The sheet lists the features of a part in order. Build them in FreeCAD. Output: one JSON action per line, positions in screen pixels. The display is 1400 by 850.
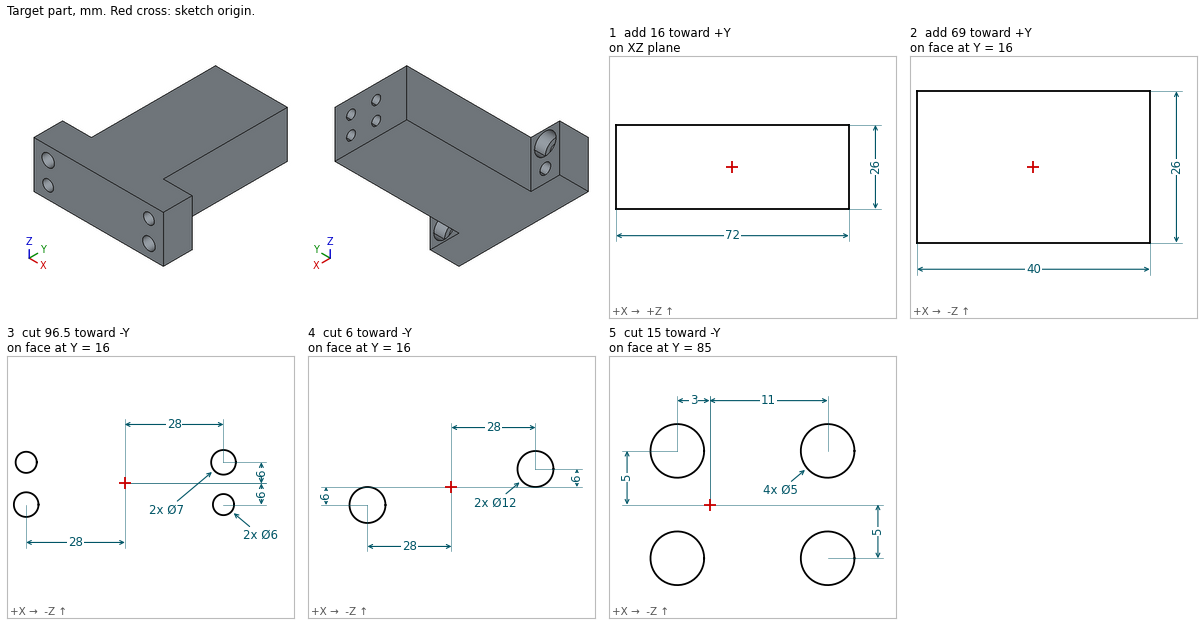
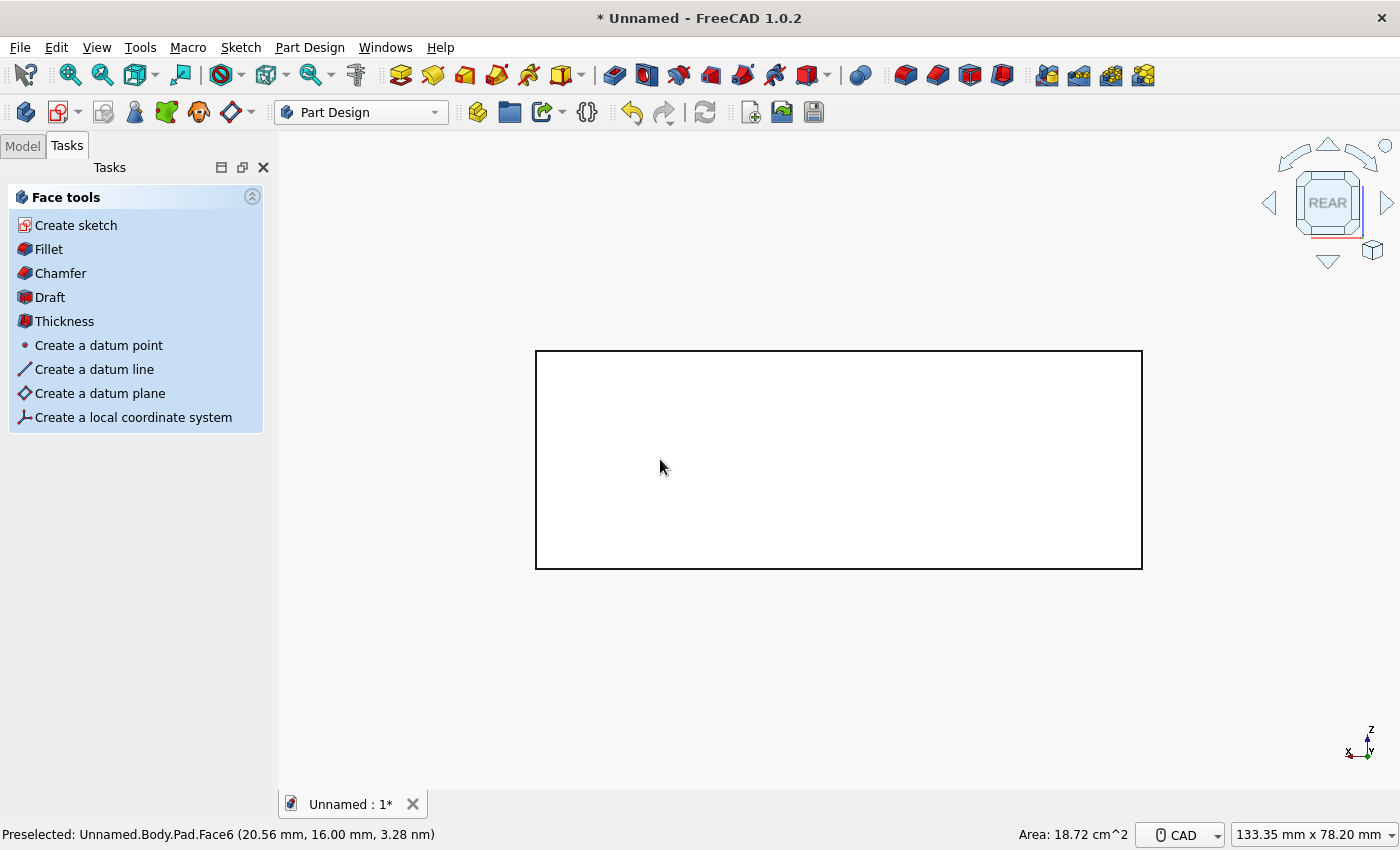
{"action": "left_click", "coordinate": [58, 112]}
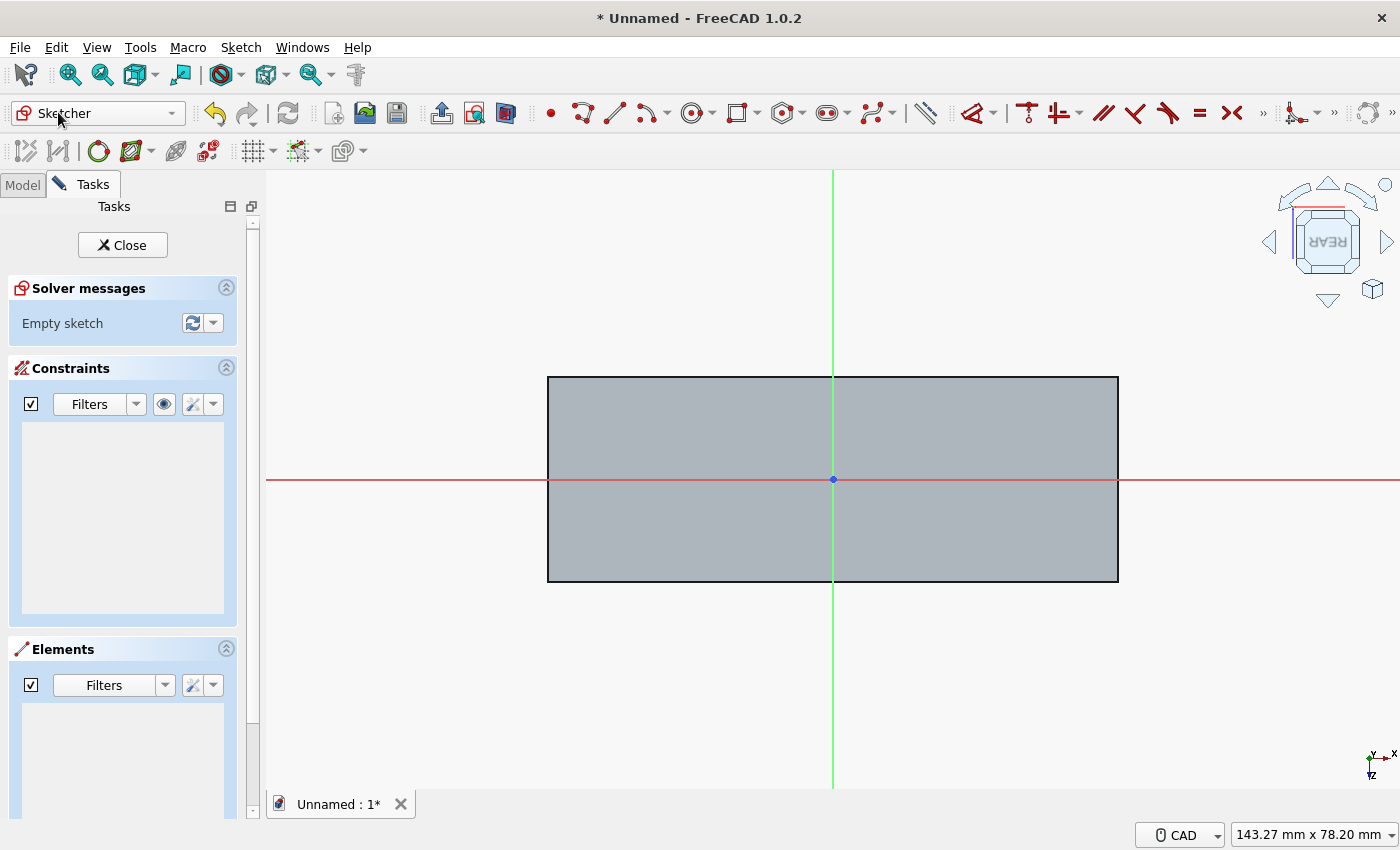
{"action": "scroll", "coordinate": [916, 479], "scroll_direction": "up", "scroll_amount": 3}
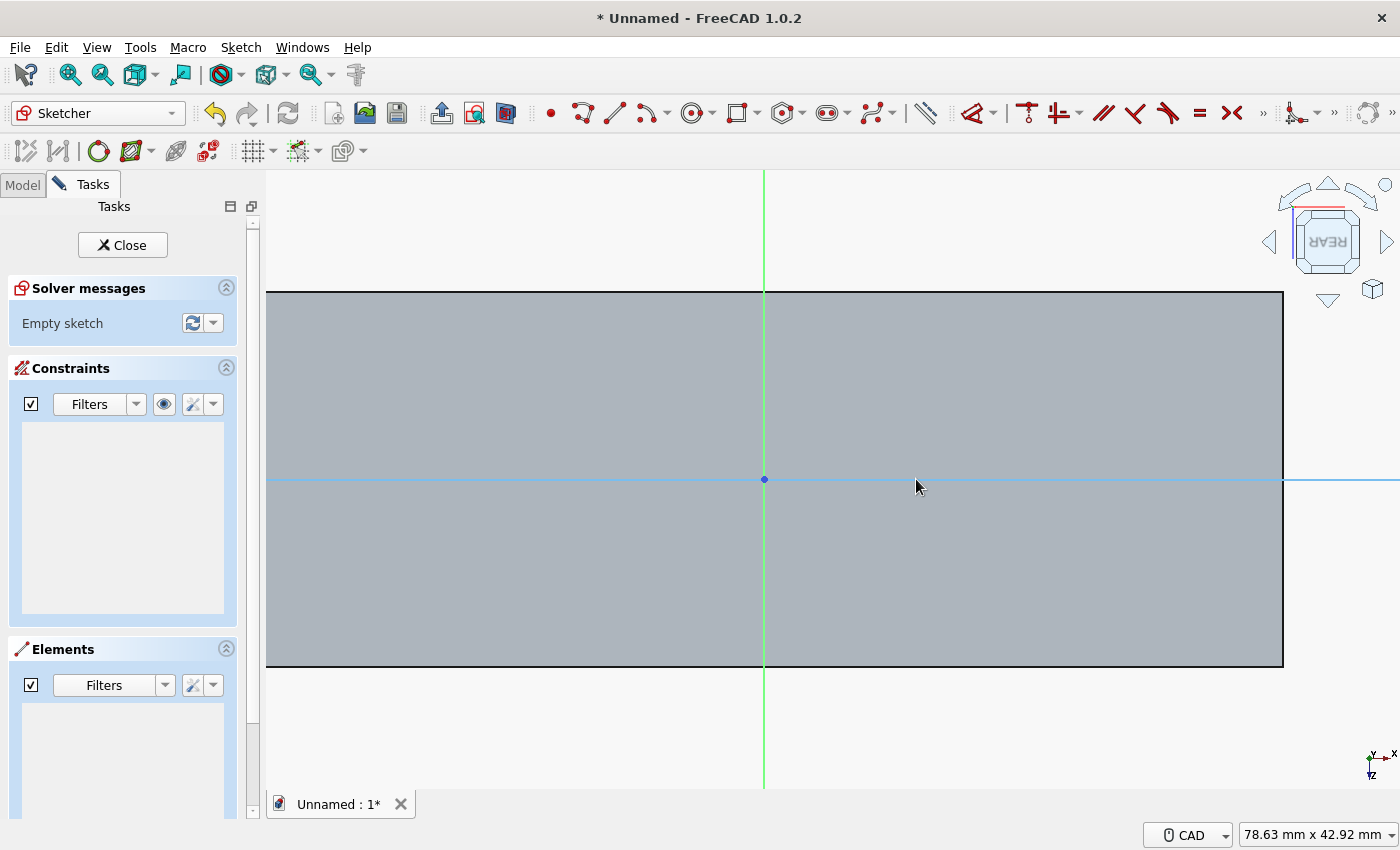
{"action": "key", "text": "g v"}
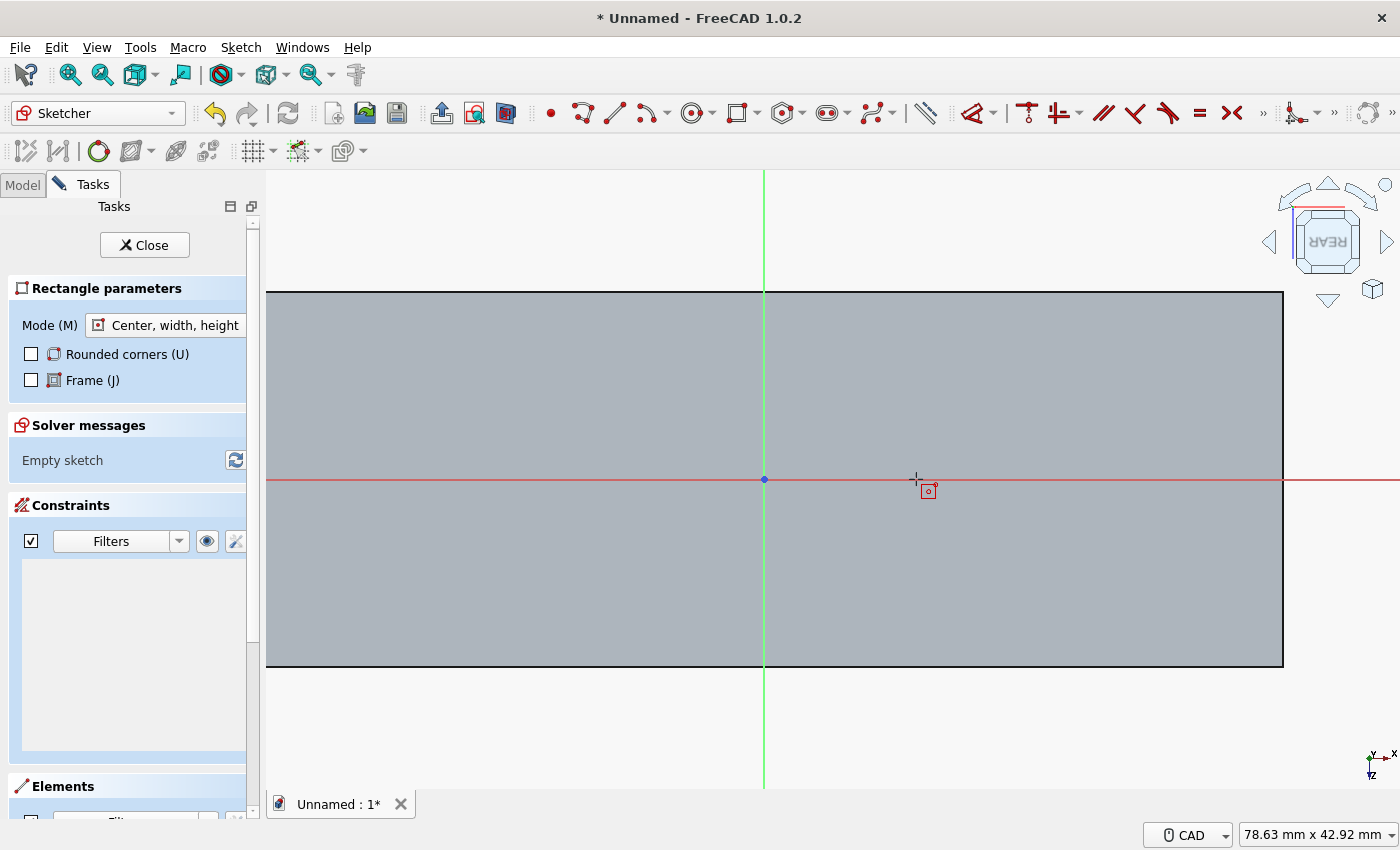
{"action": "left_click", "coordinate": [764, 479]}
{"action": "mouse_move", "coordinate": [1053, 292]}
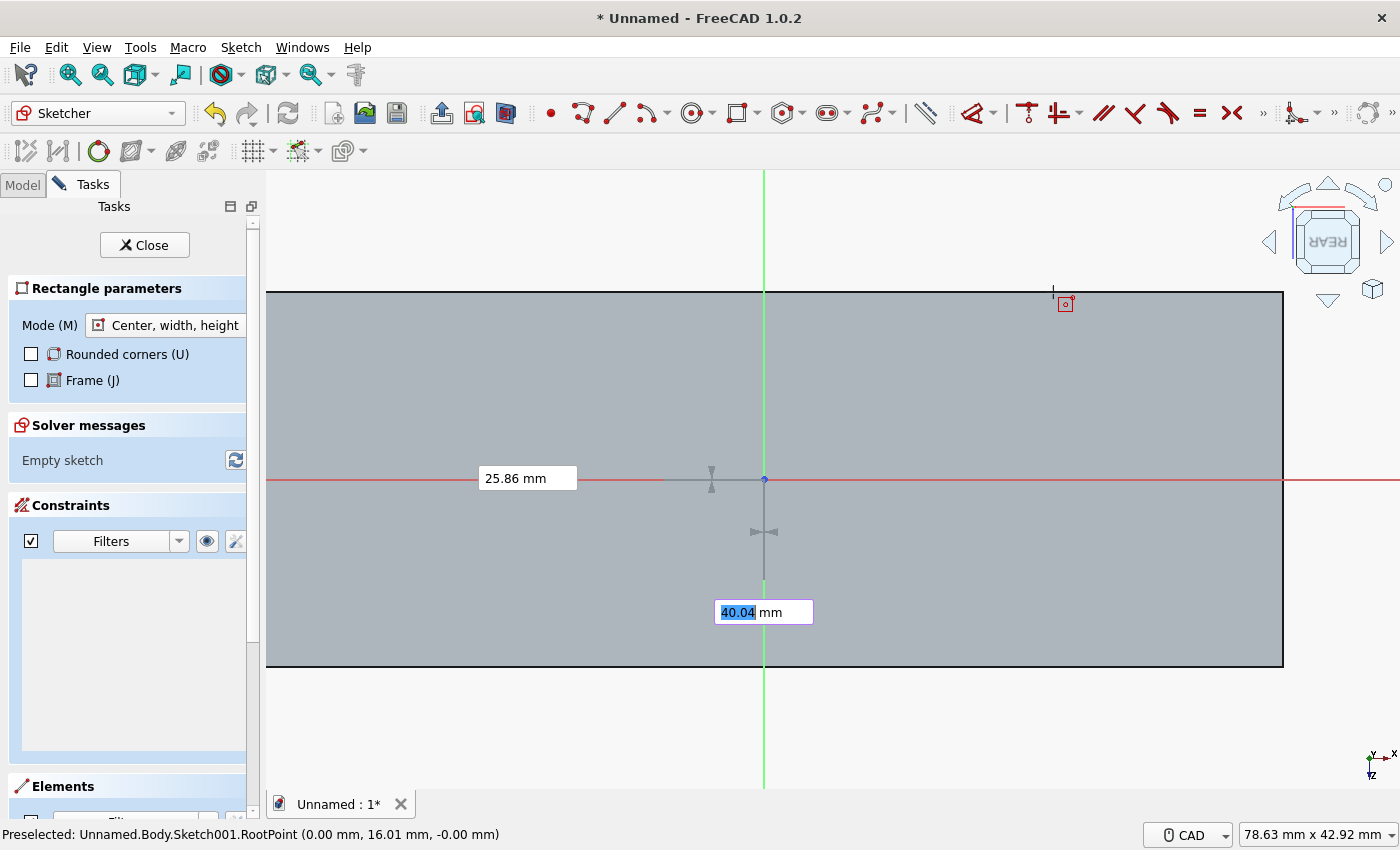
{"action": "type", "text": "40"}
{"action": "key", "text": "Tab"}
{"action": "type", "text": "26"}
{"action": "key", "text": "Return"}
{"action": "key", "text": "Escape"}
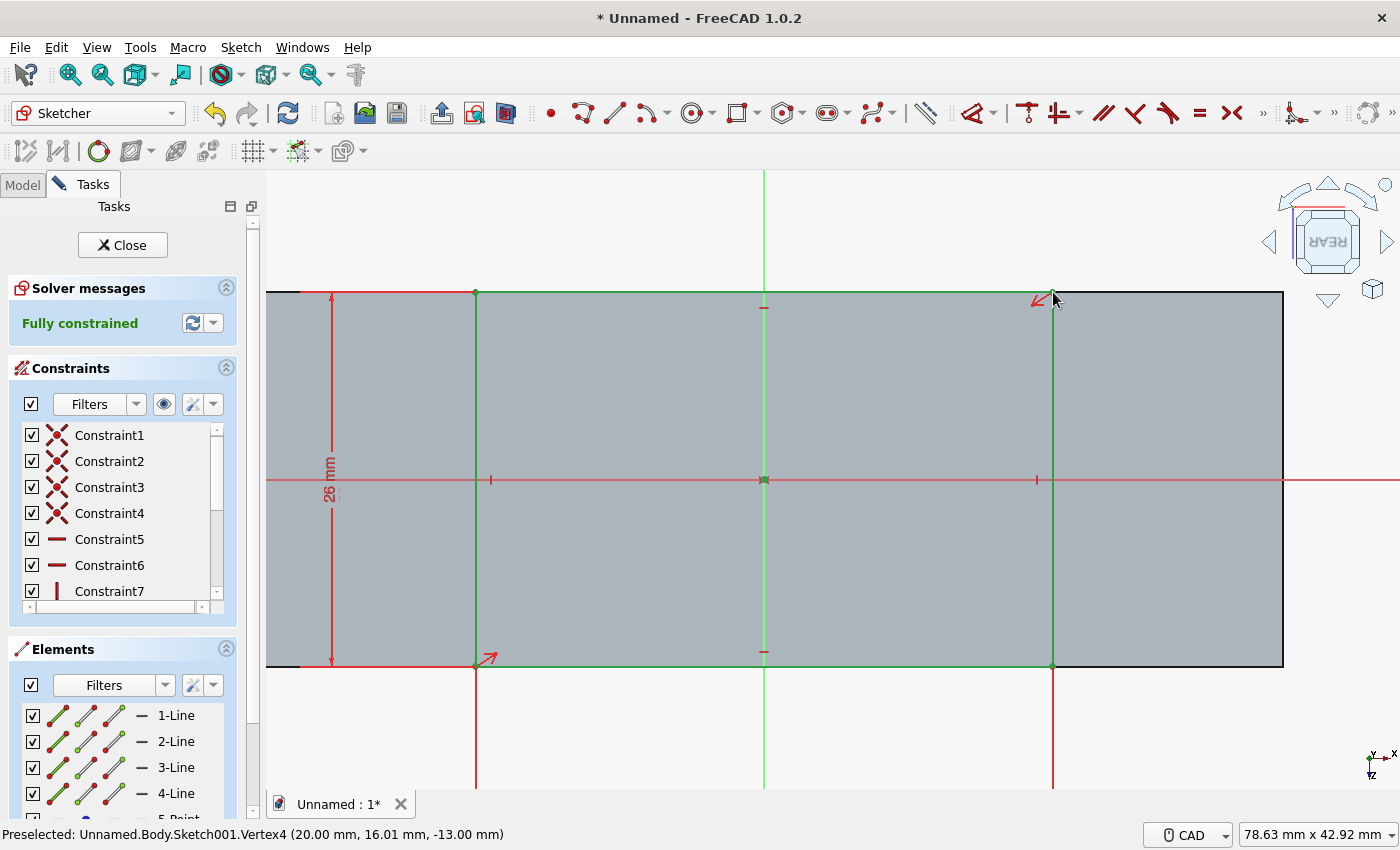
{"action": "left_click", "coordinate": [123, 245]}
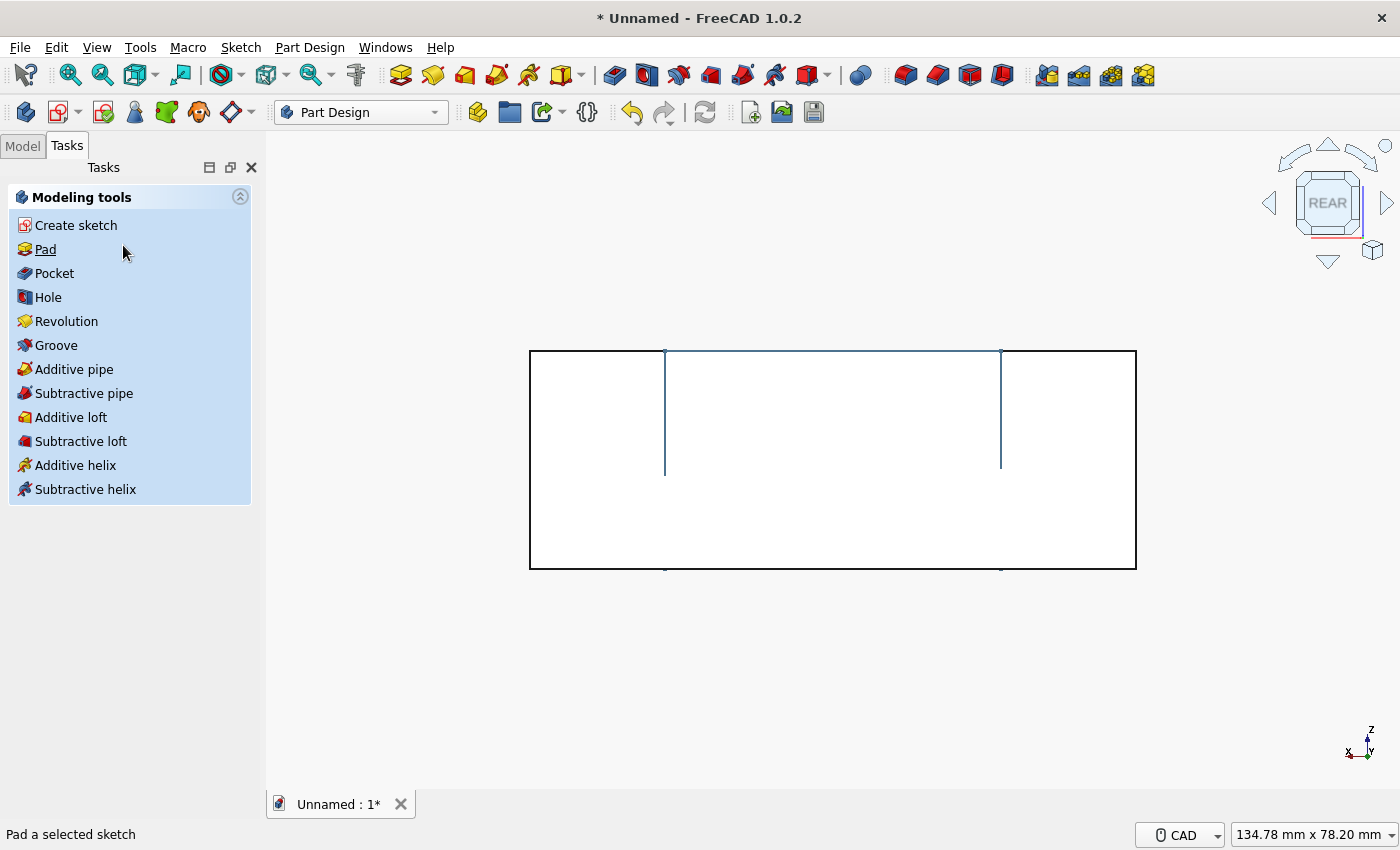
{"action": "left_click", "coordinate": [402, 76]}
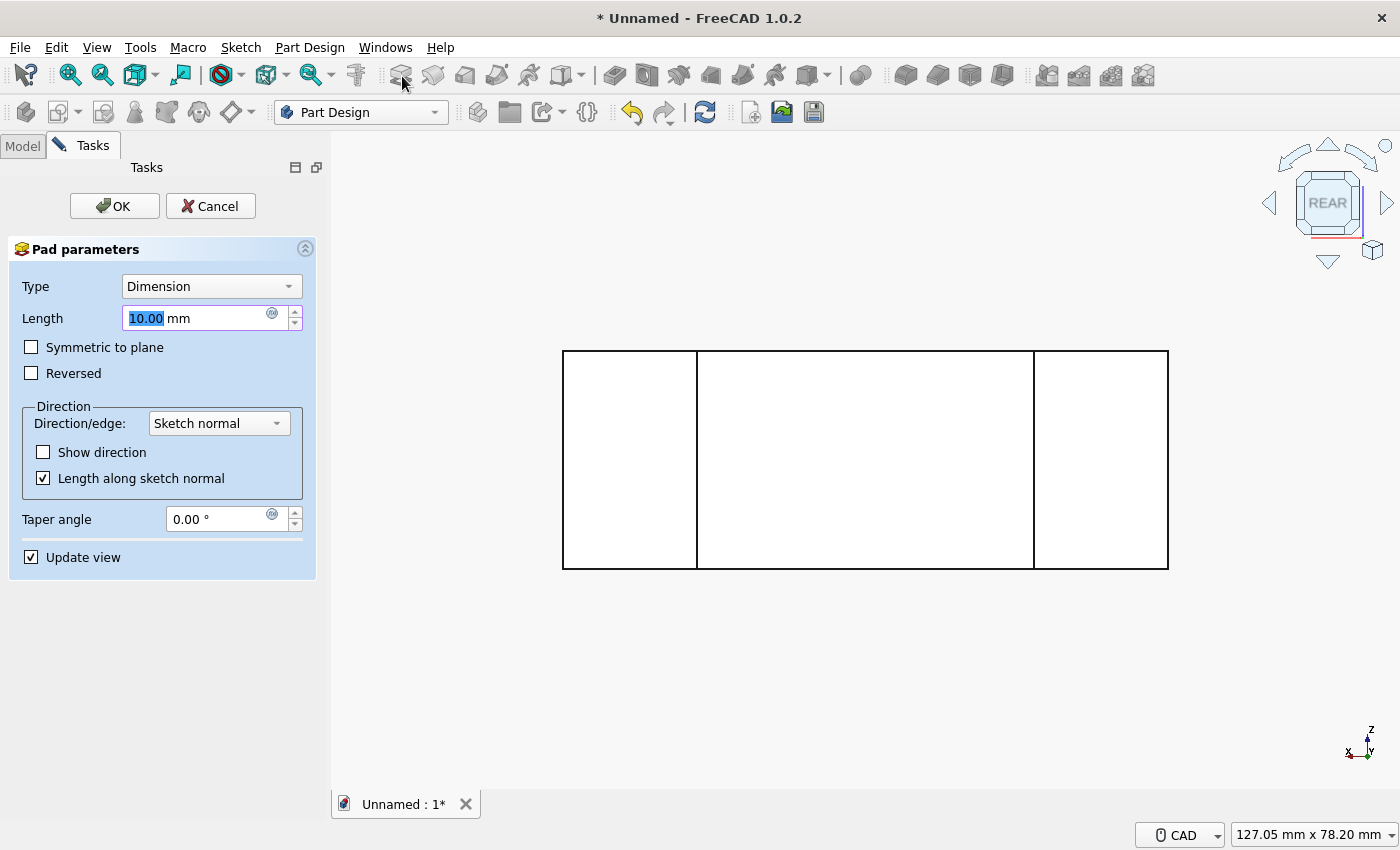
{"action": "type", "text": "69"}
{"action": "key", "text": "Tab"}